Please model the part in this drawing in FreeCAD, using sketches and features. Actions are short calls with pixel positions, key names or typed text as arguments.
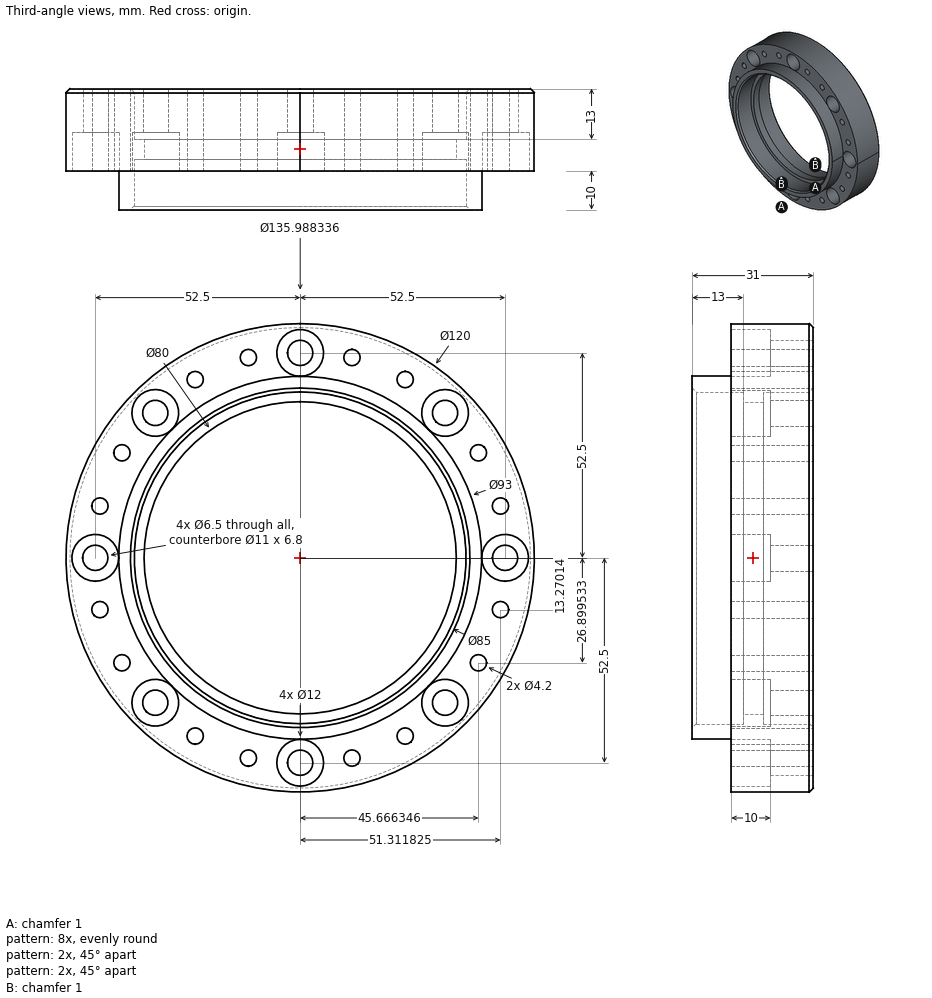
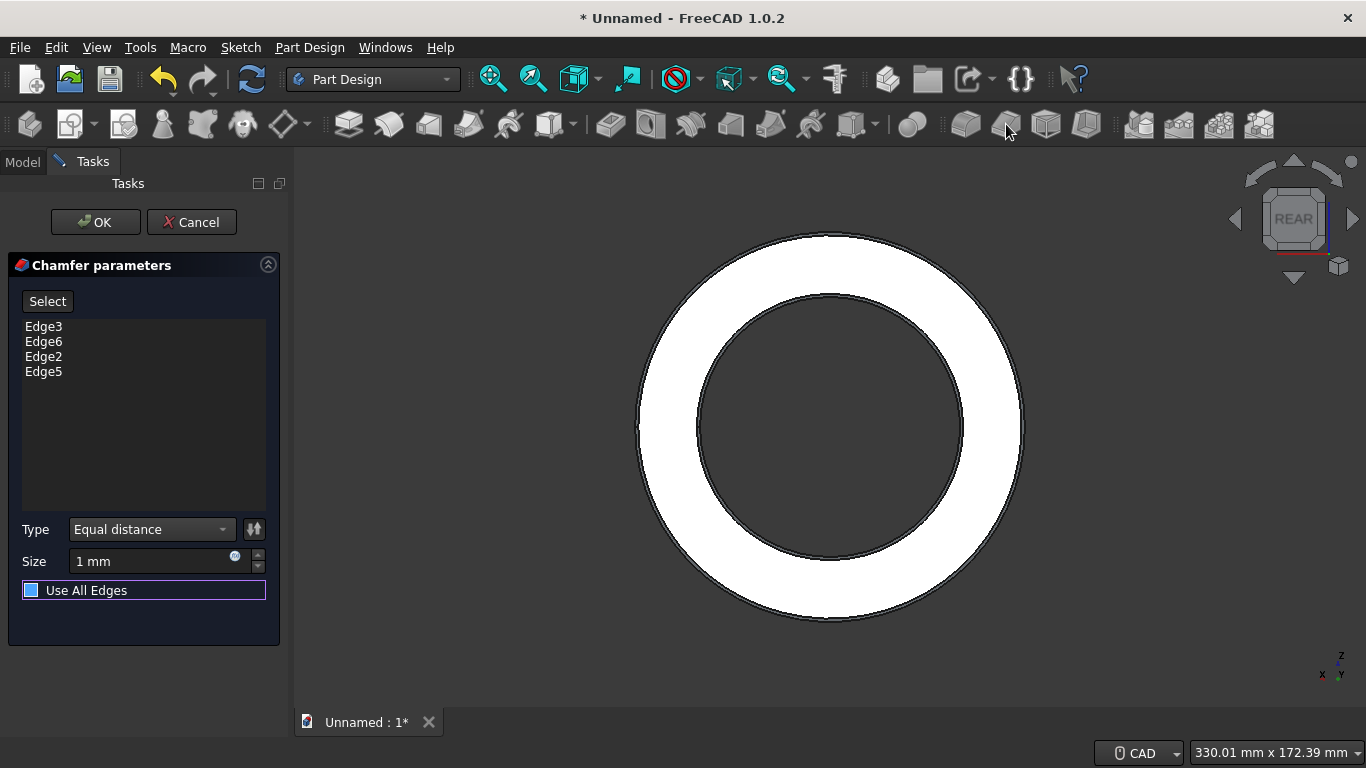
click(96, 222)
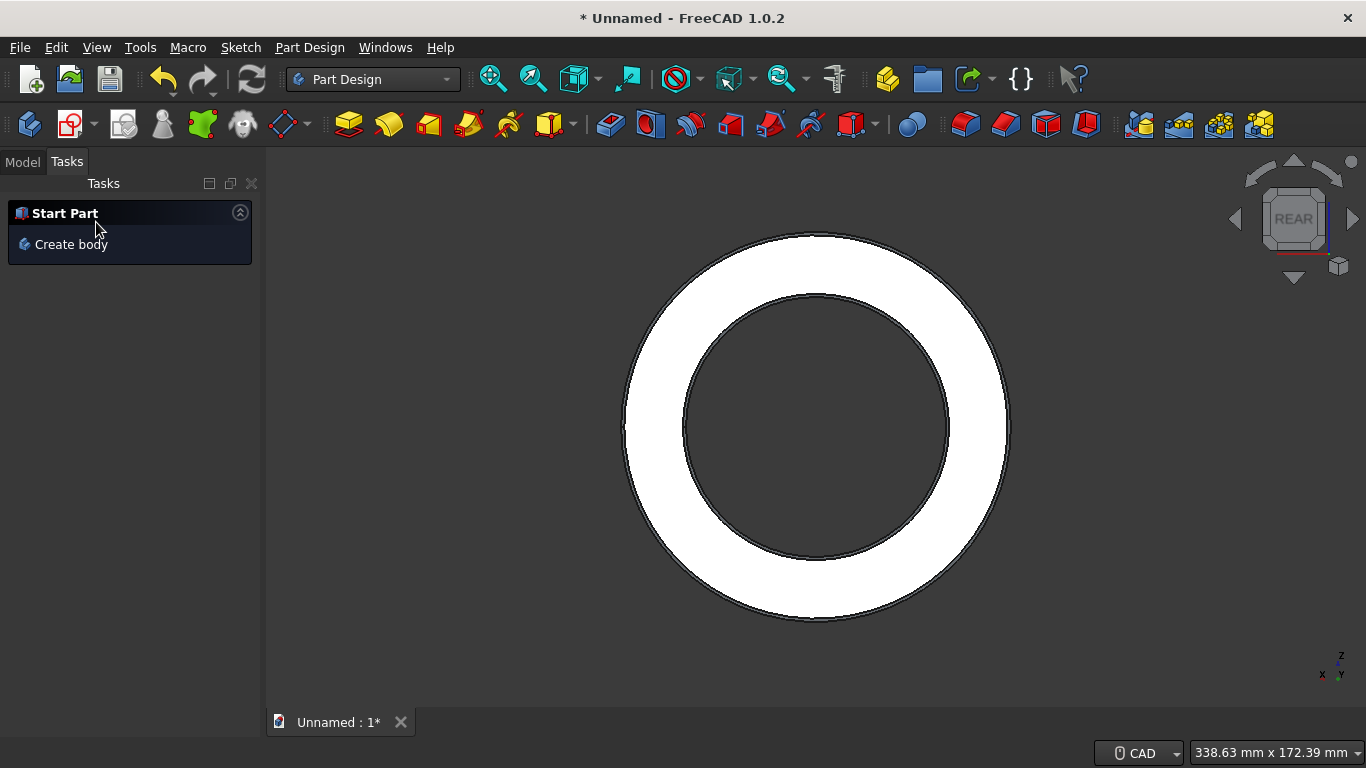
key(0)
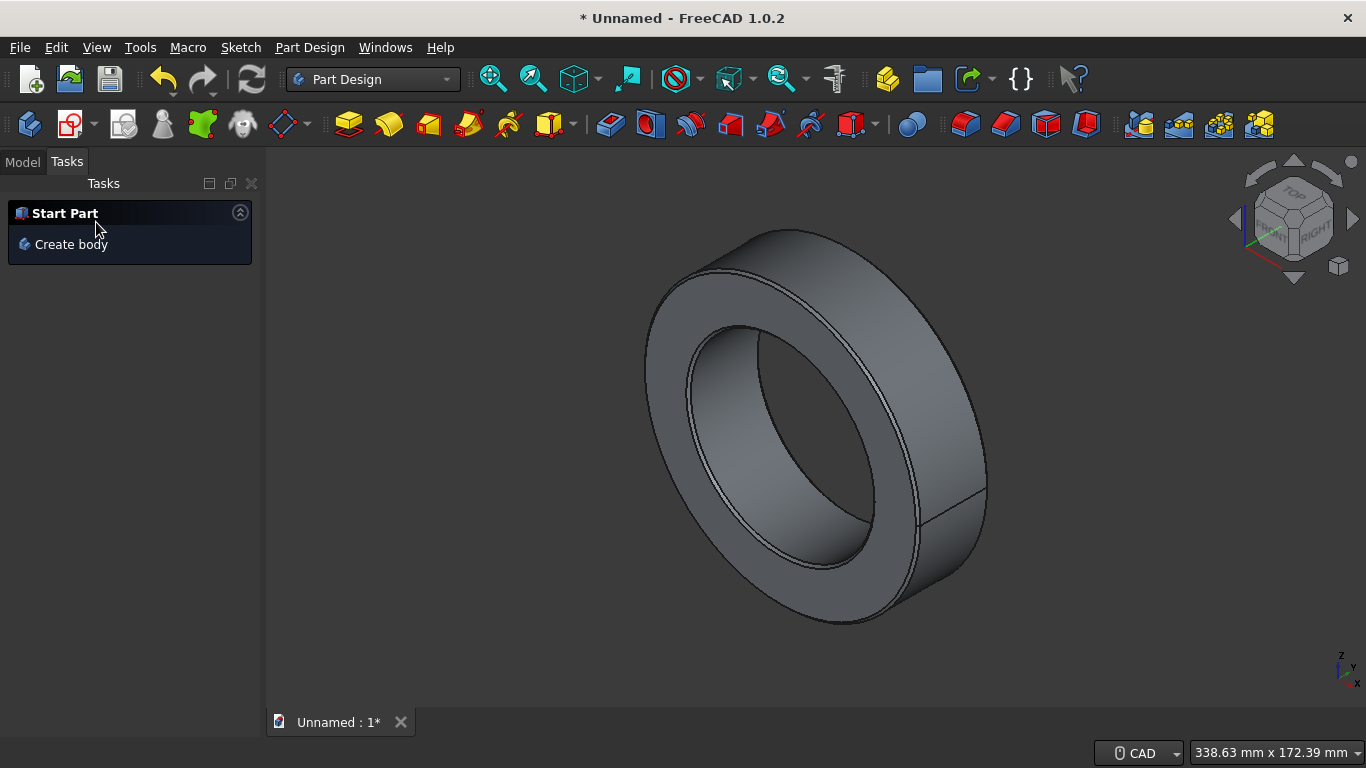
click(780, 312)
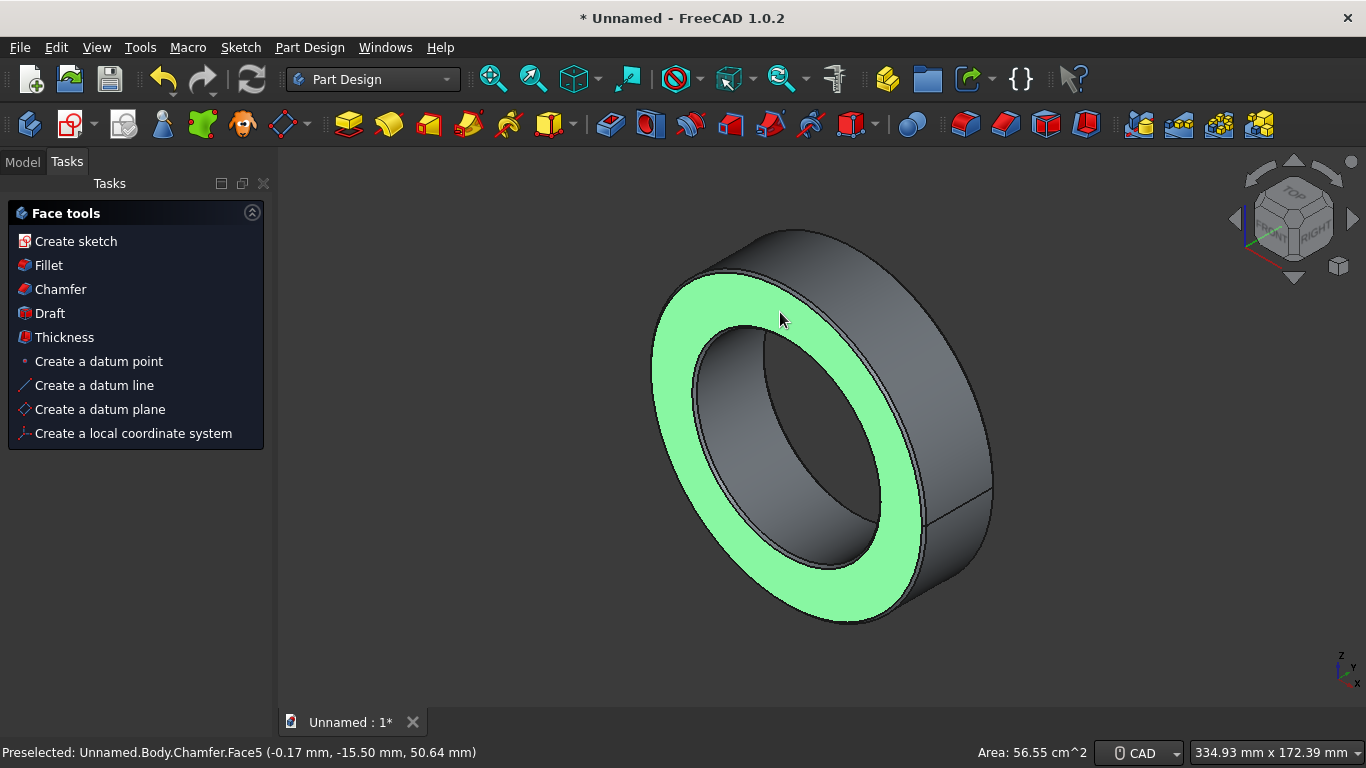
click(70, 124)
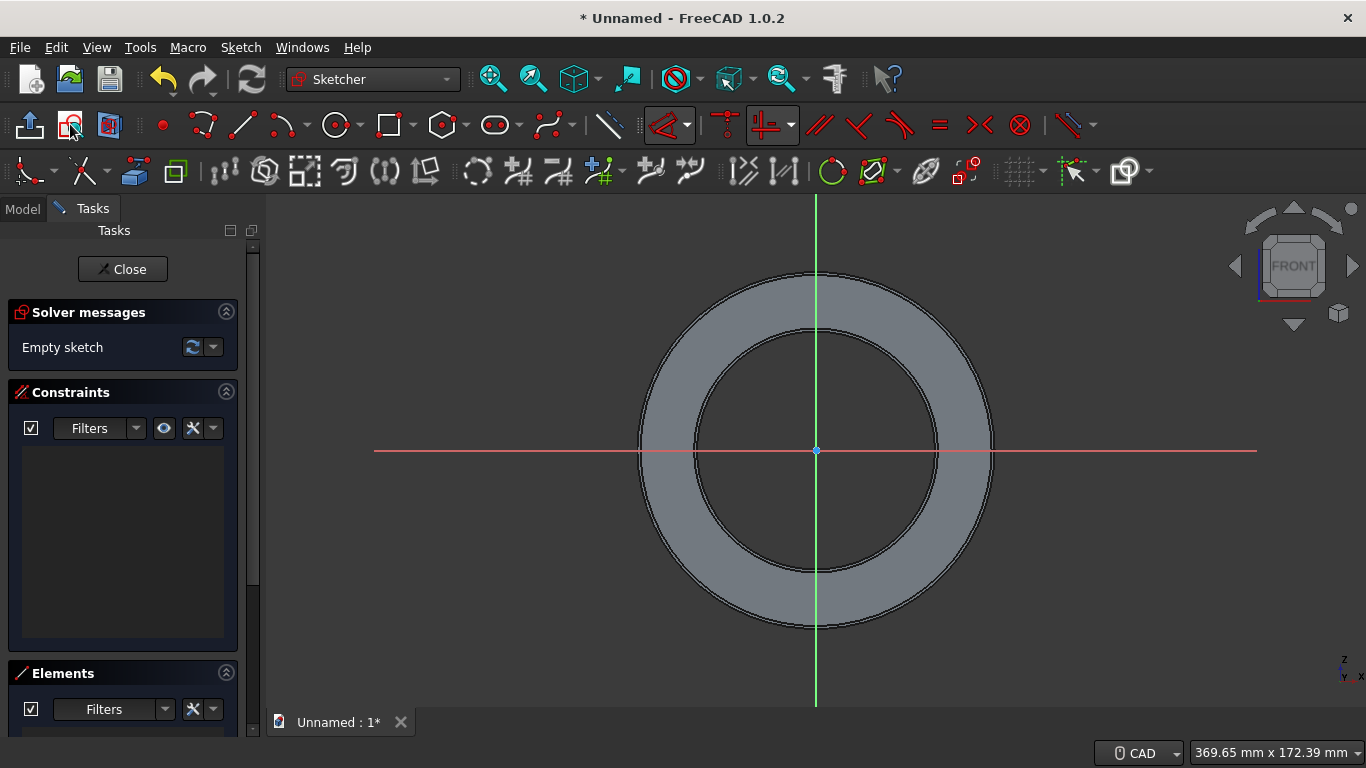
click(336, 126)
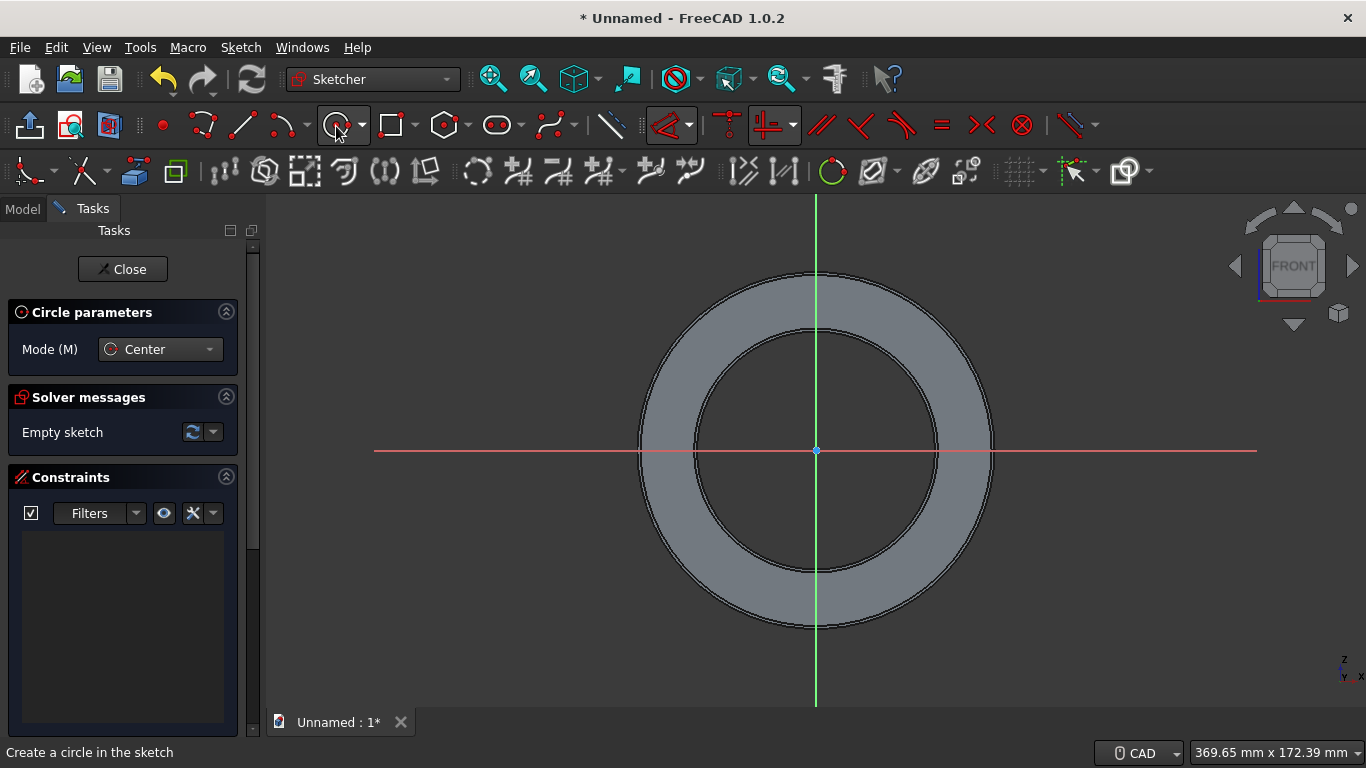
scroll(660, 450, up, 5)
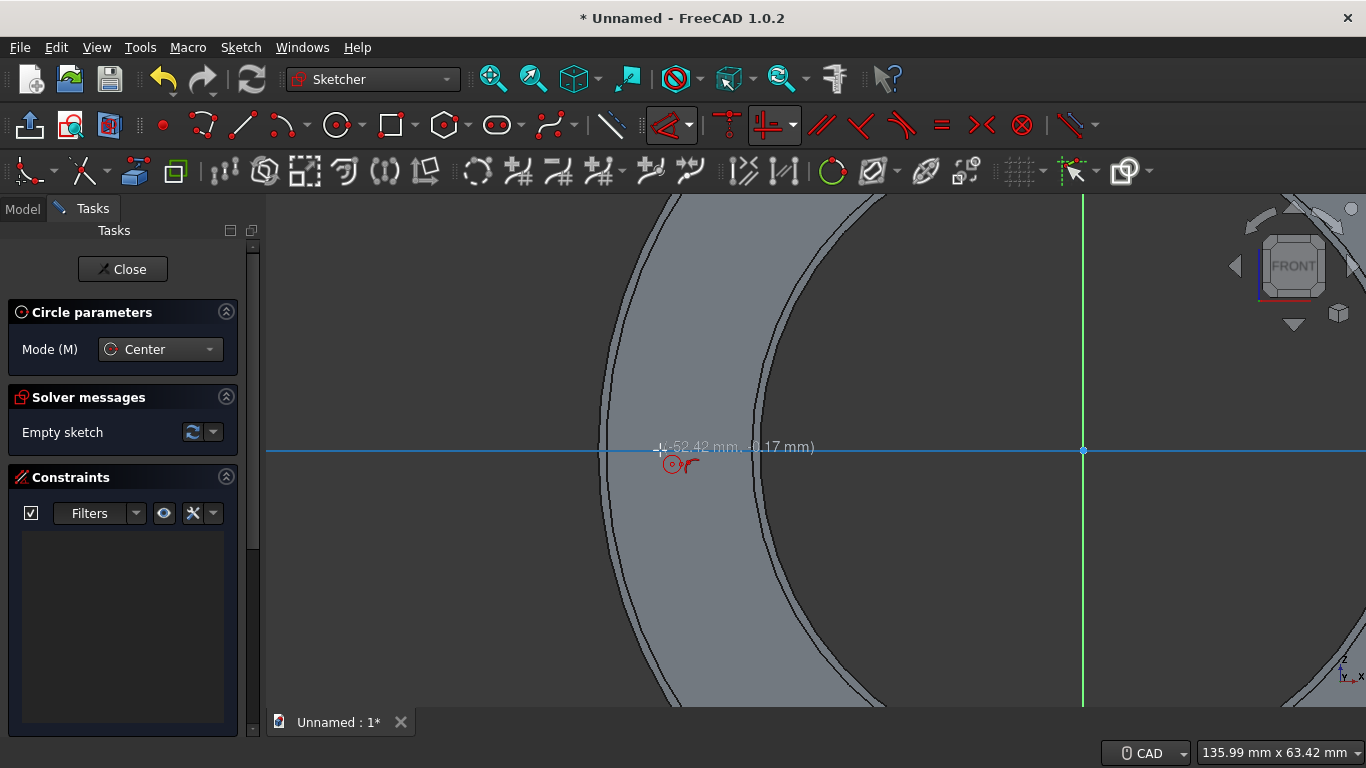
click(659, 450)
move(677, 432)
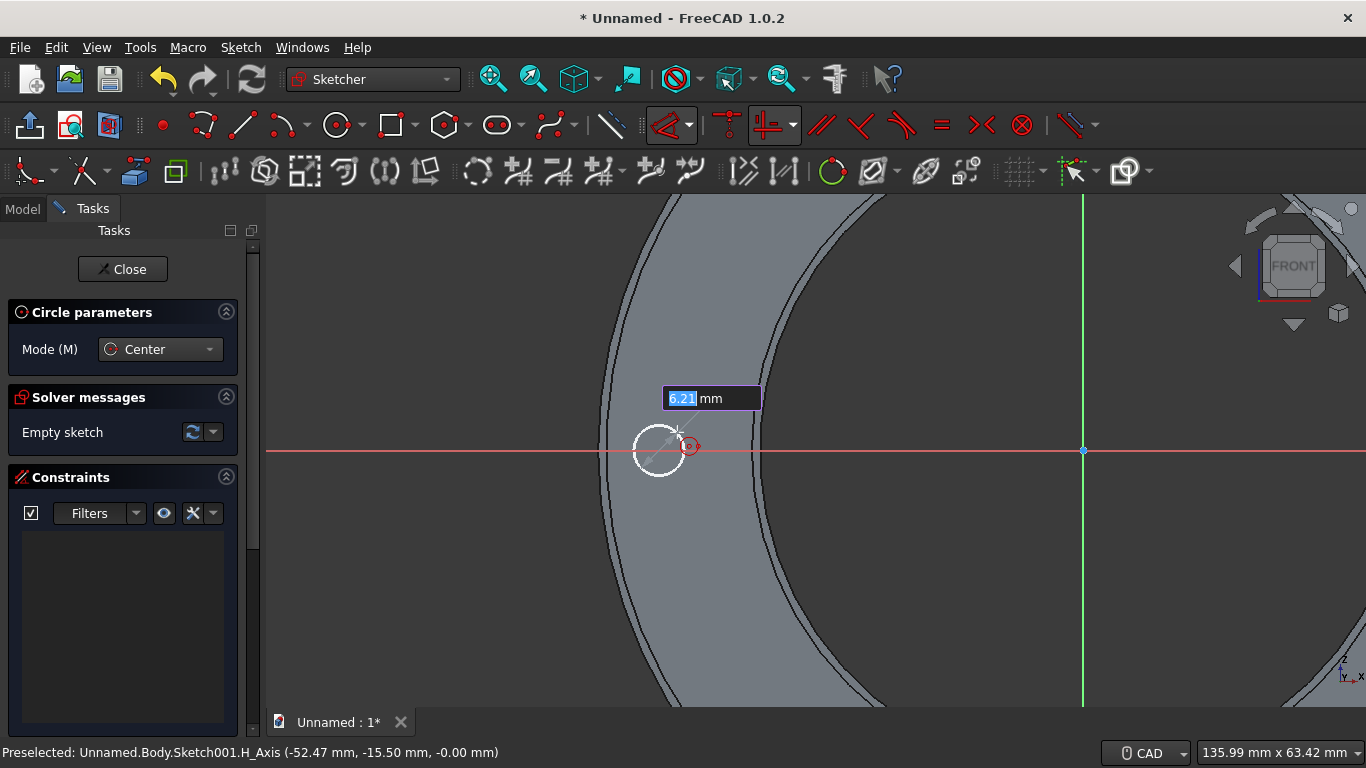
text(6.5)
key(Return)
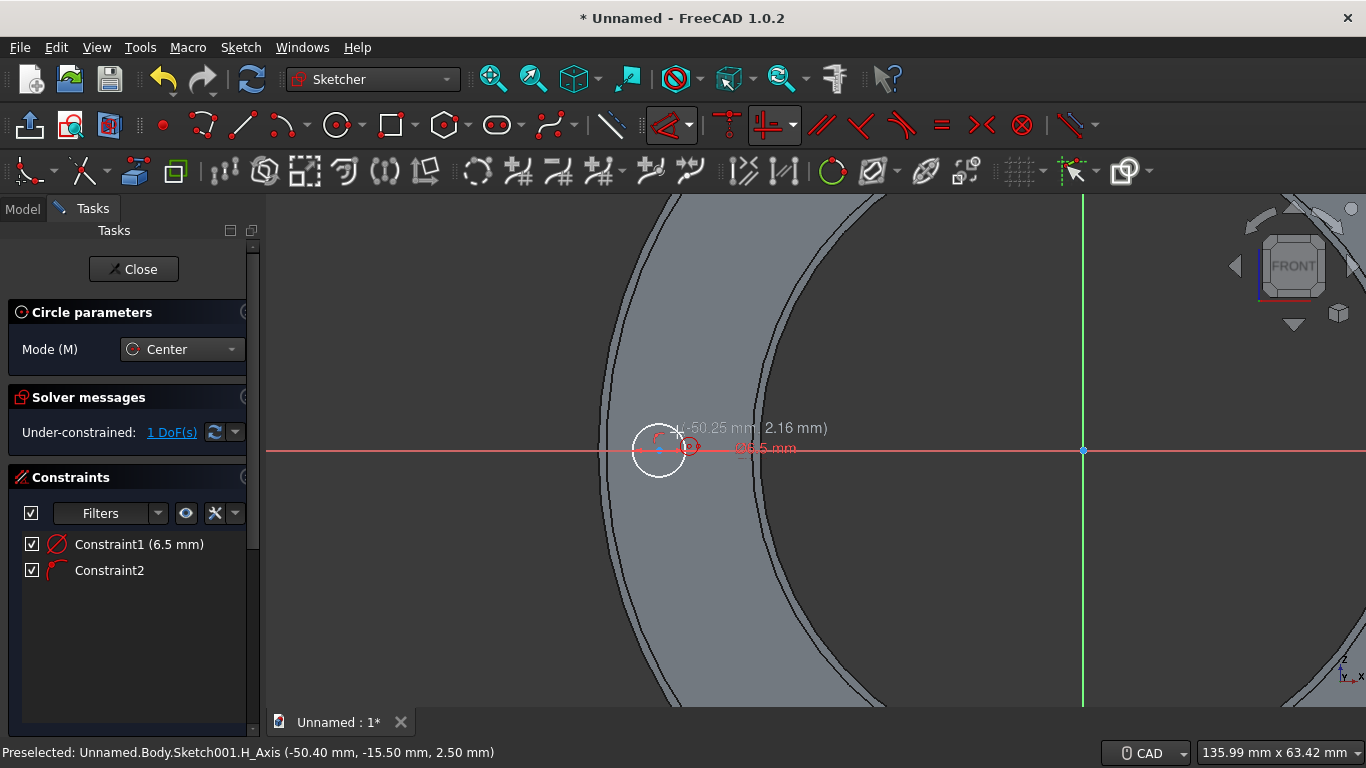
scroll(552, 451, down, 5)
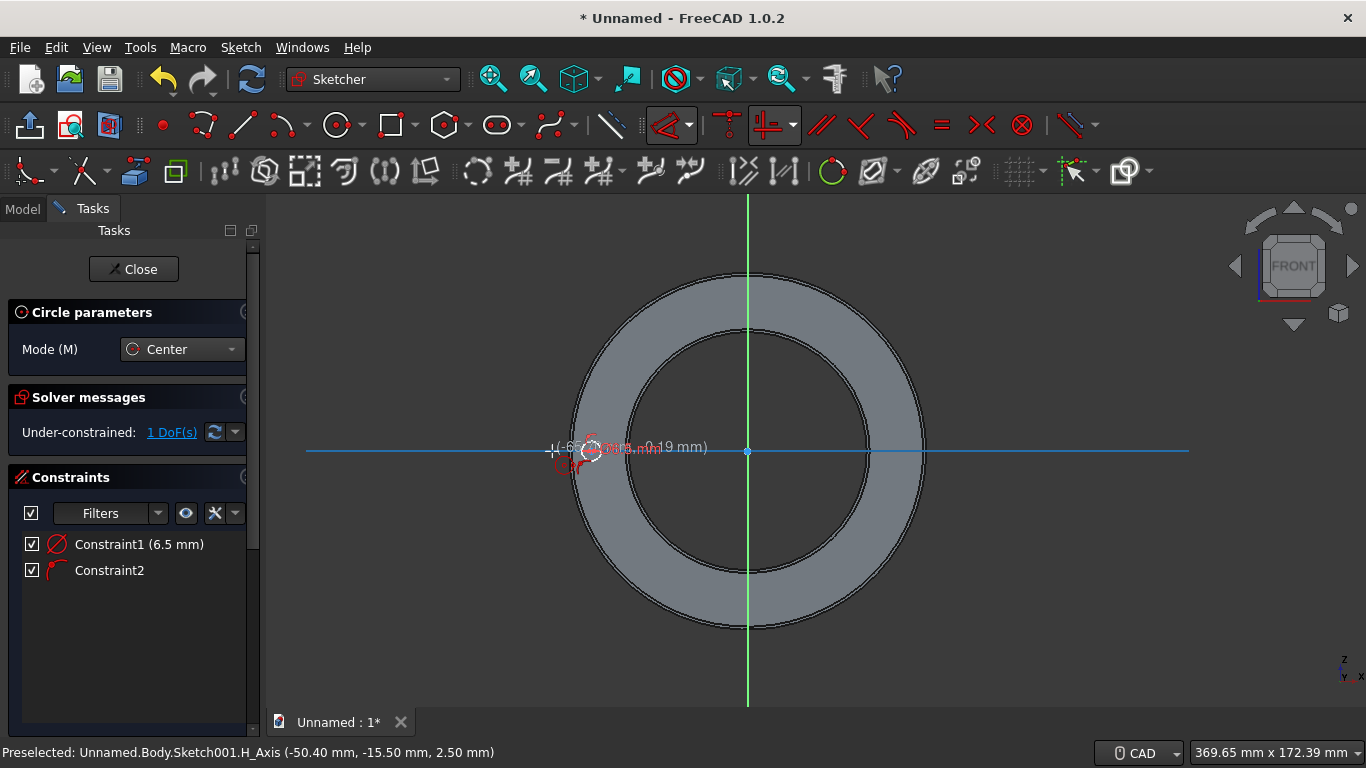
scroll(904, 451, up, 5)